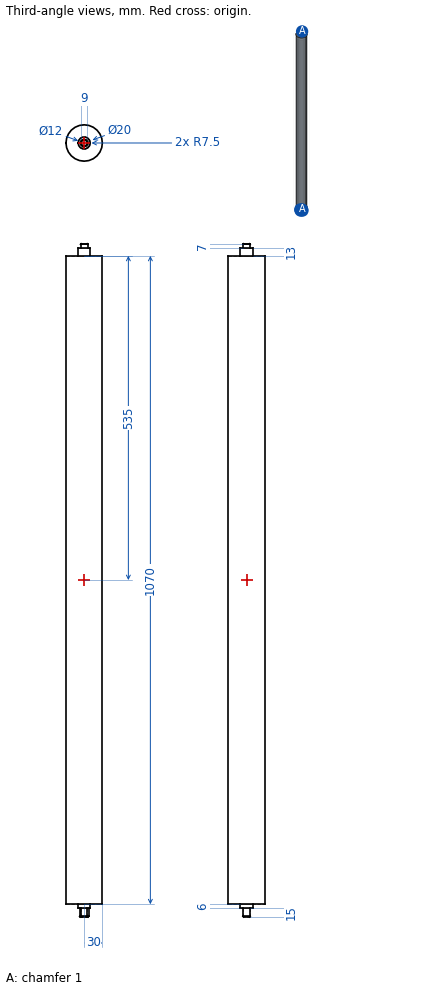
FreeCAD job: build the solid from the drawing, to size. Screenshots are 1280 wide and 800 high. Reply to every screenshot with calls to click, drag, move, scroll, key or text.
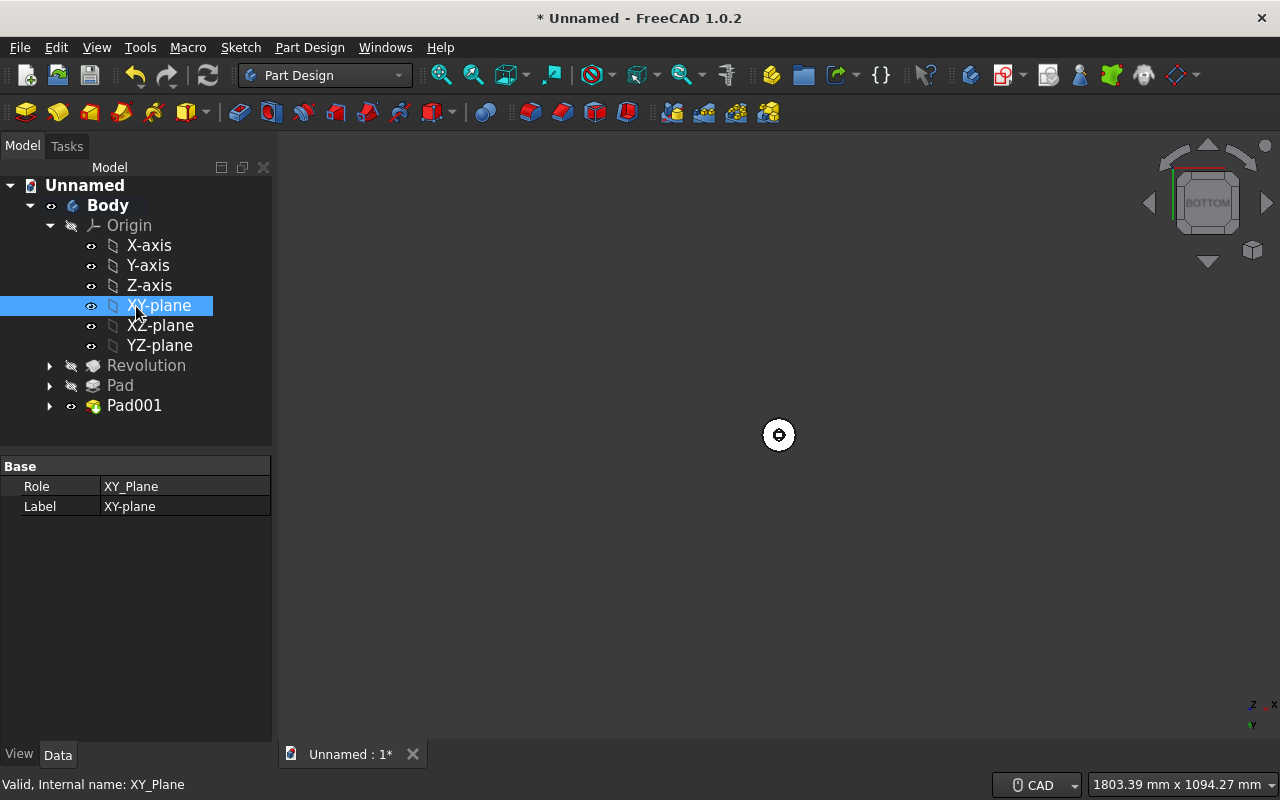
click(1176, 76)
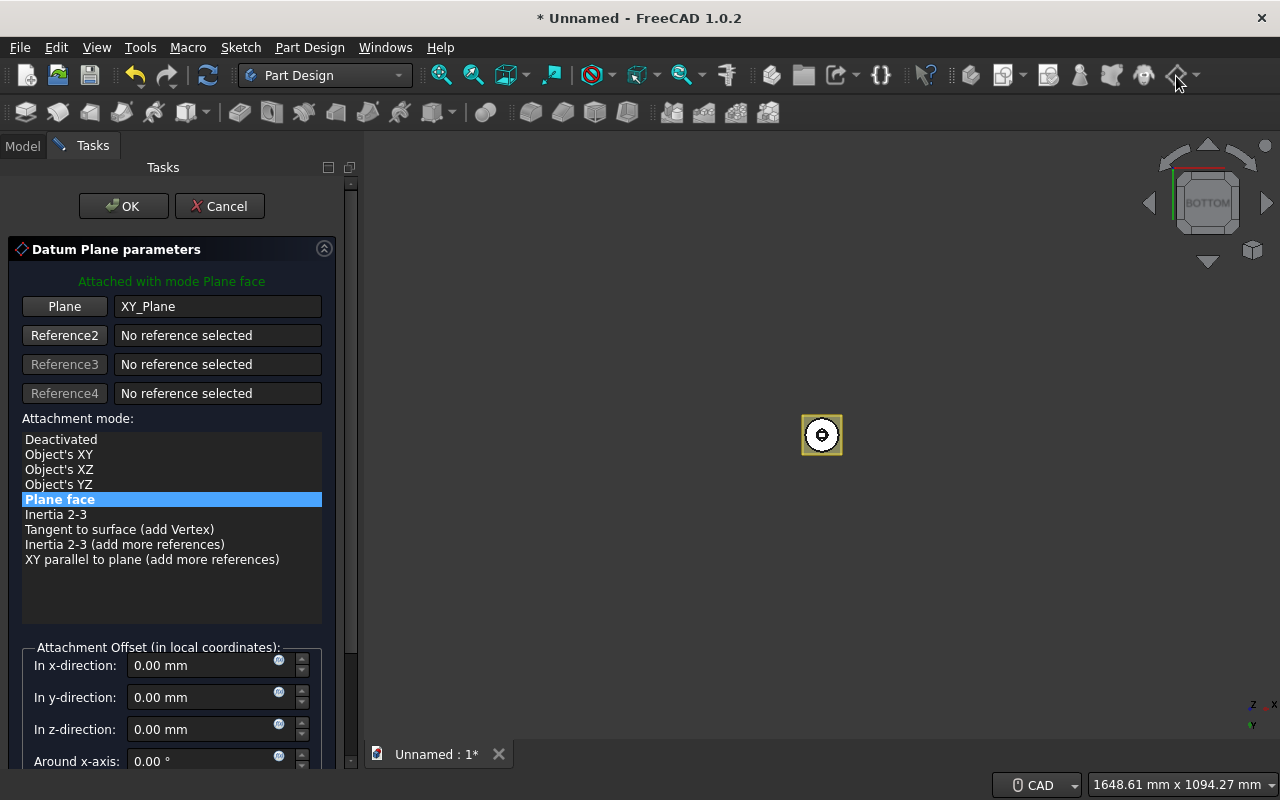
triple_click(210, 729)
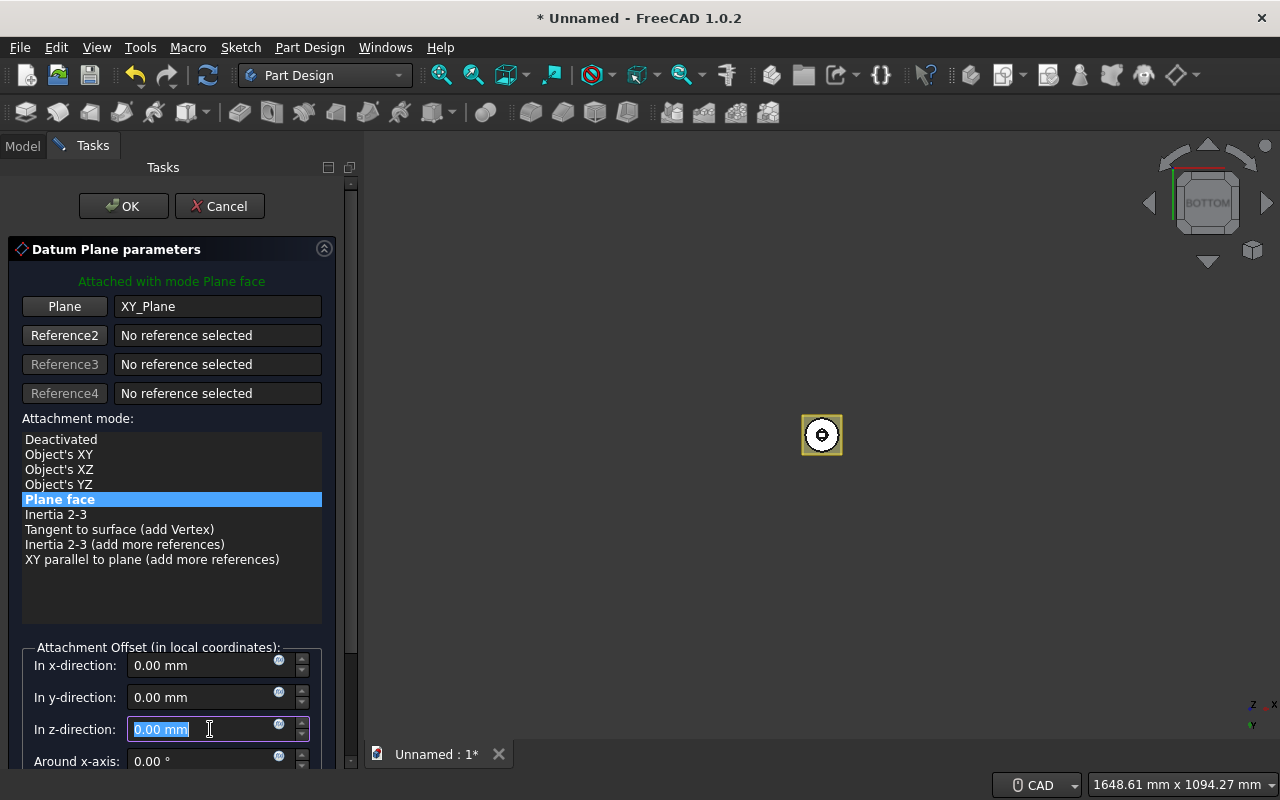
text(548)
key(Tab)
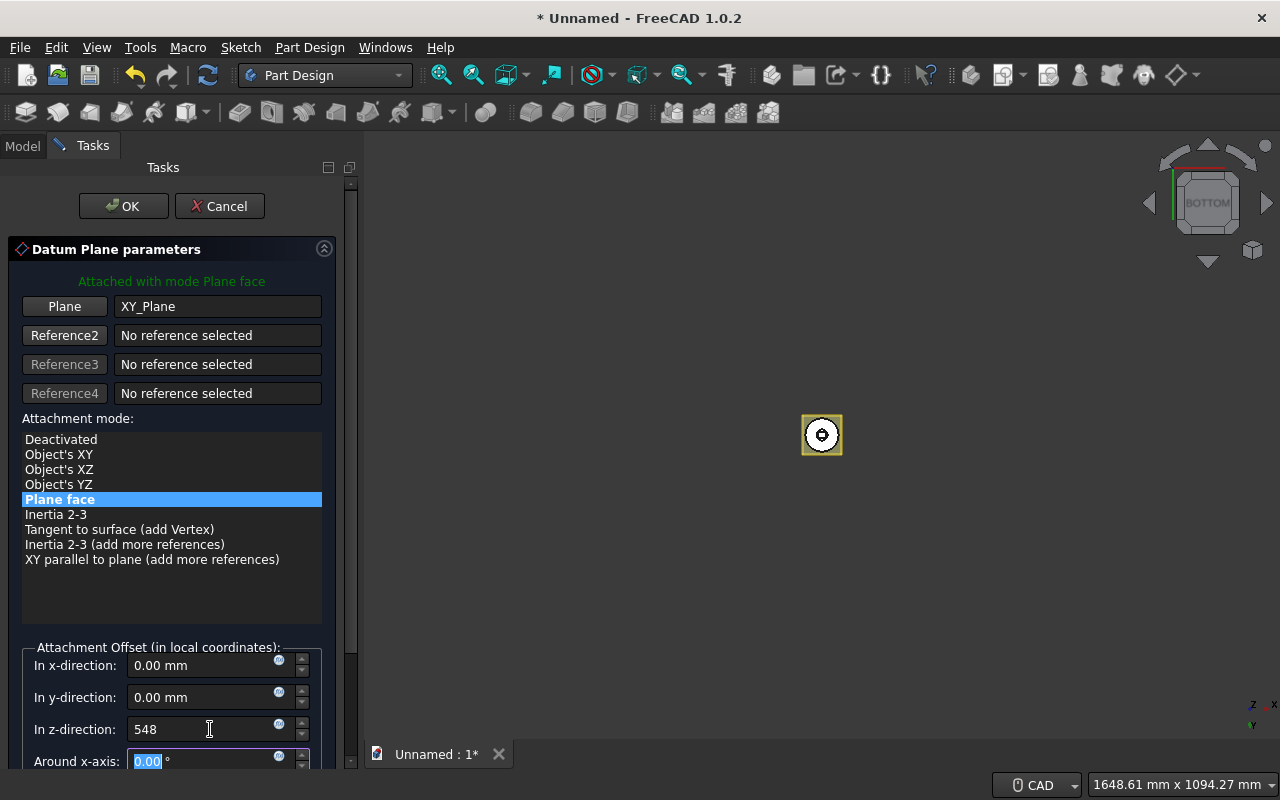
click(124, 206)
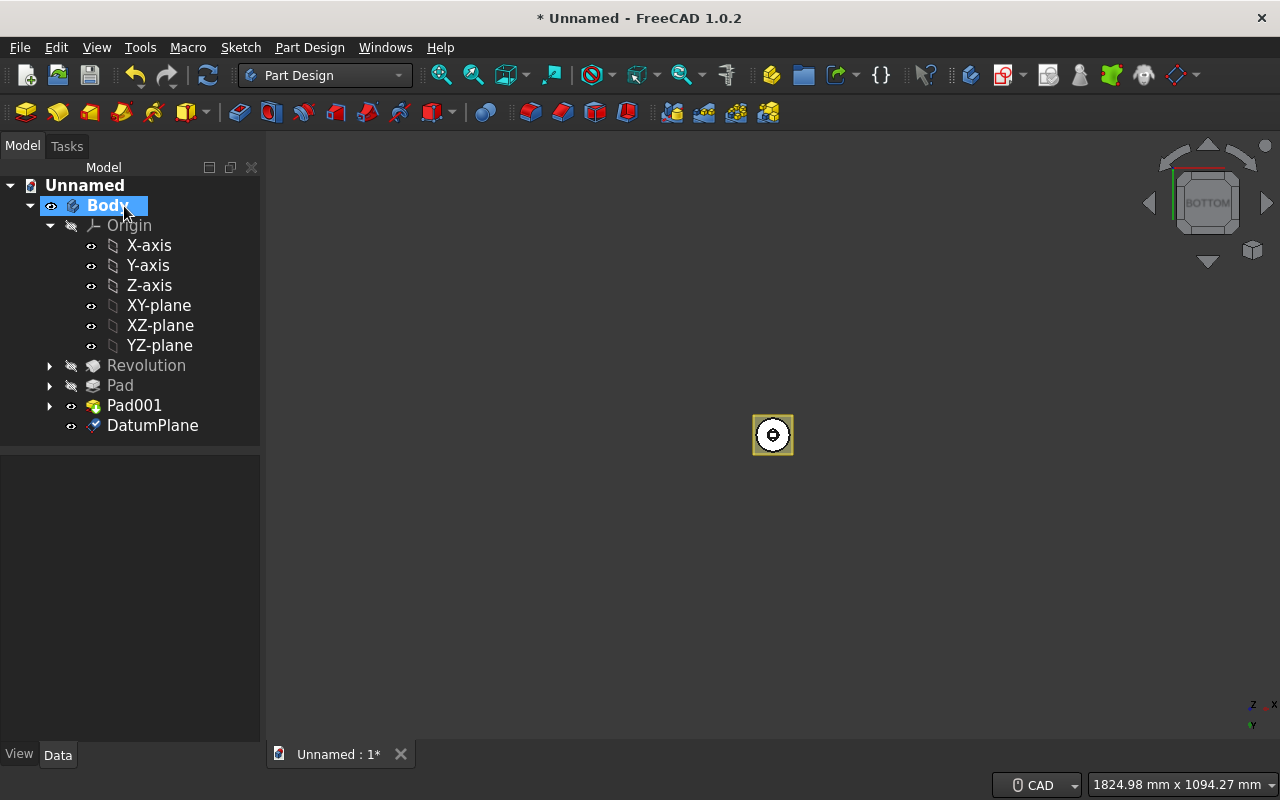
click(116, 426)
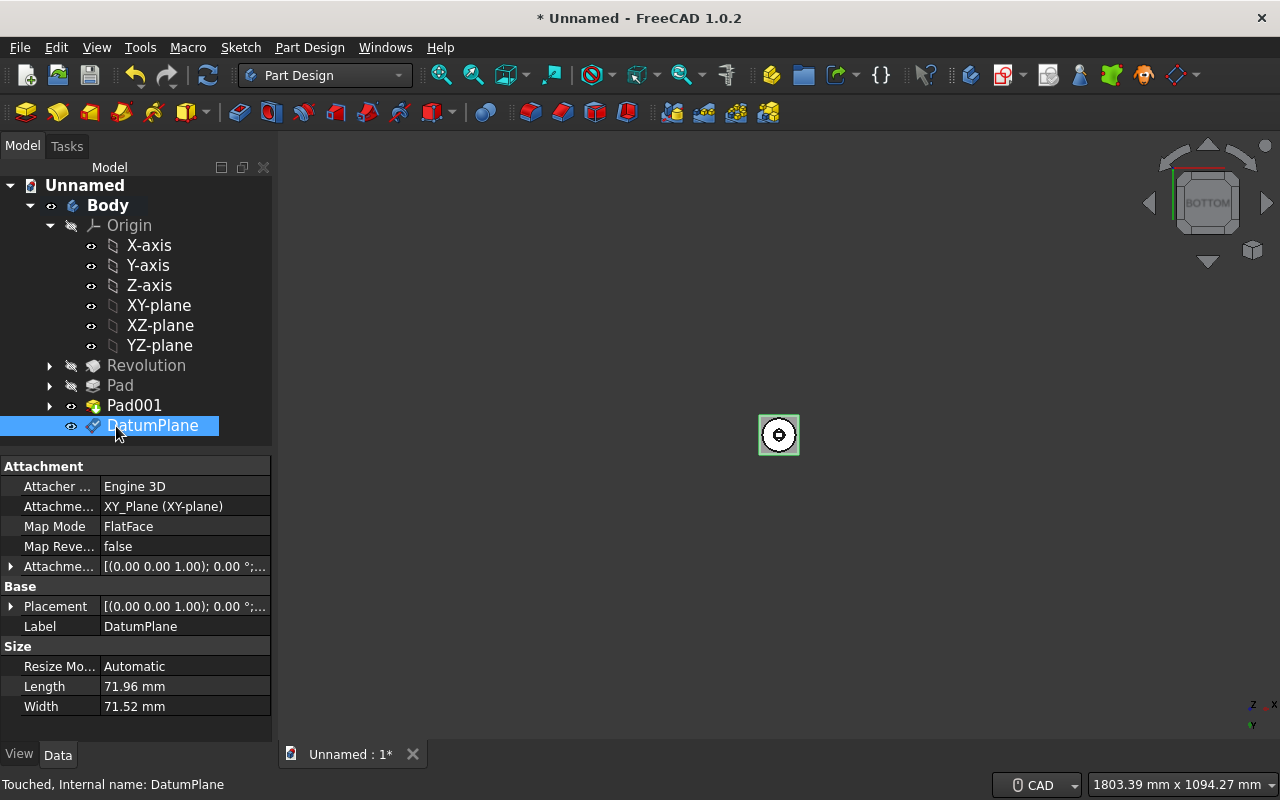
click(1004, 76)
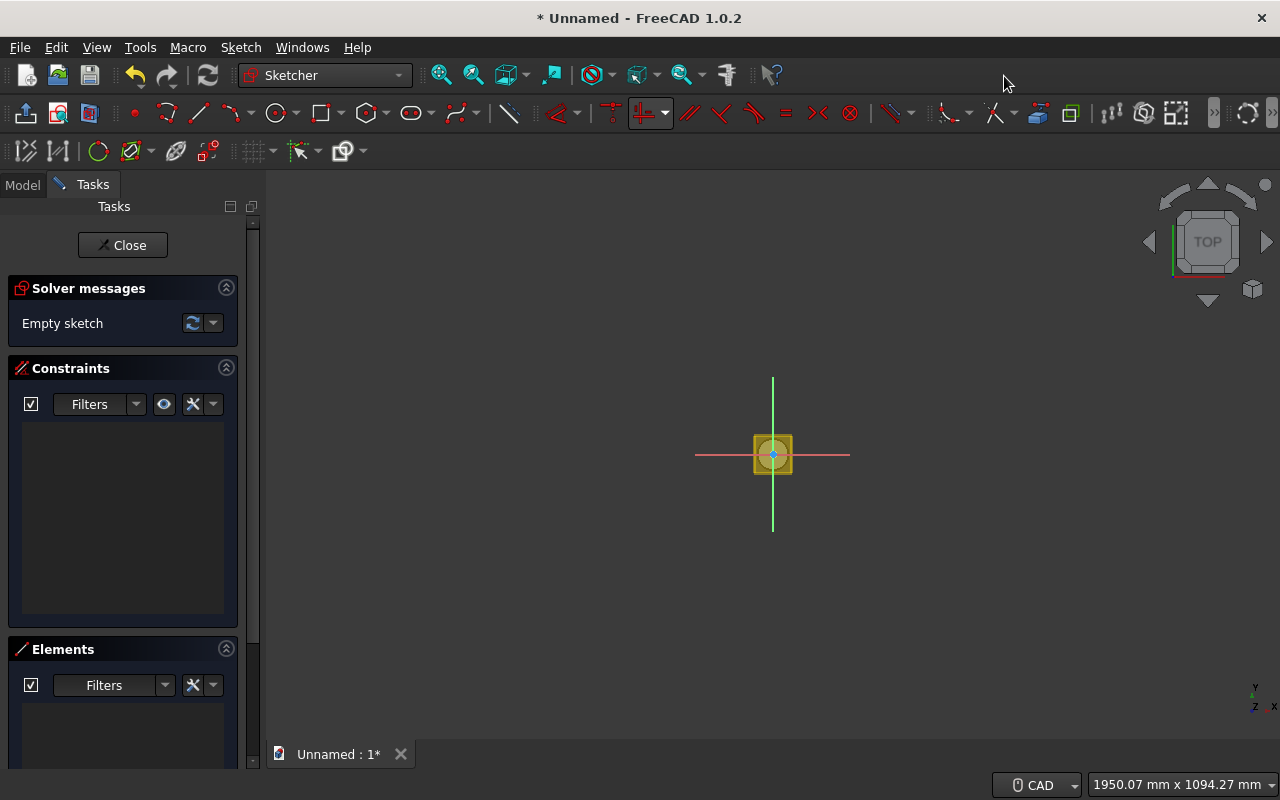
scroll(777, 455, up, 15)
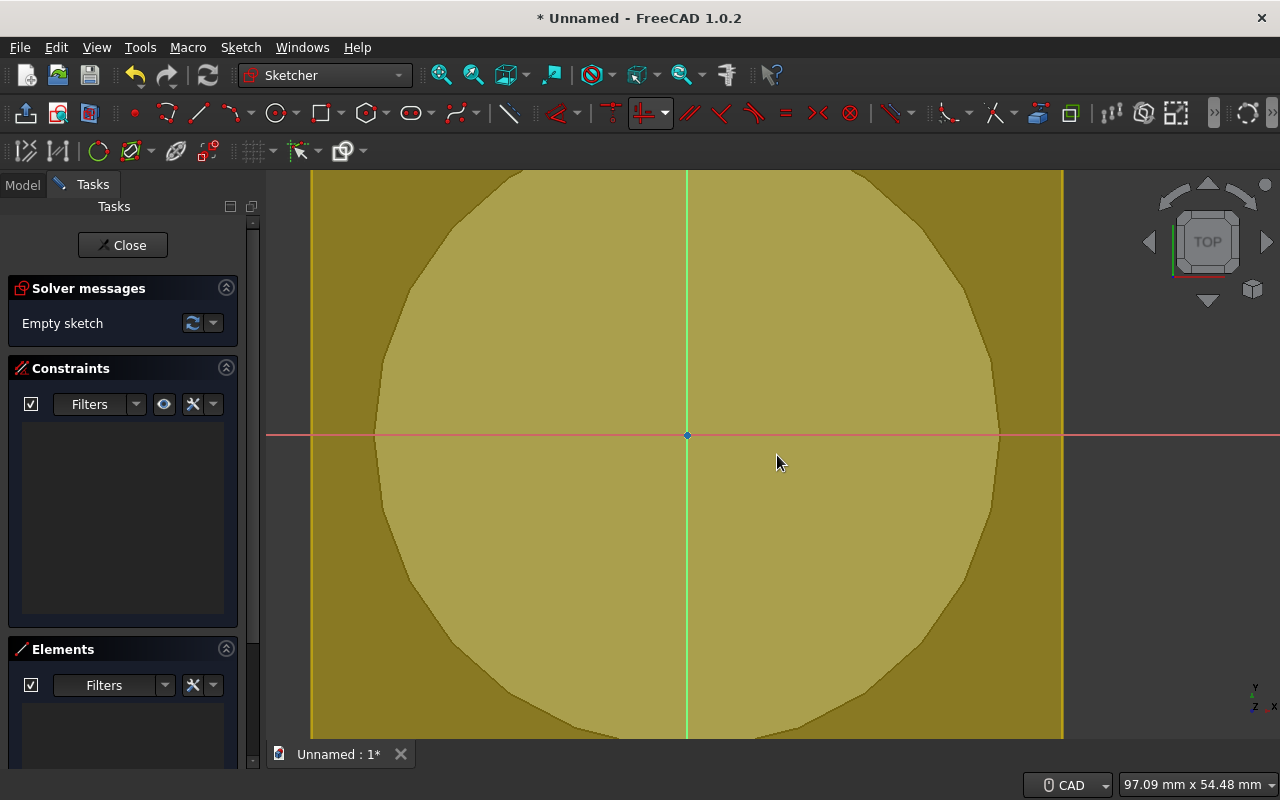
scroll(666, 412, up, 3)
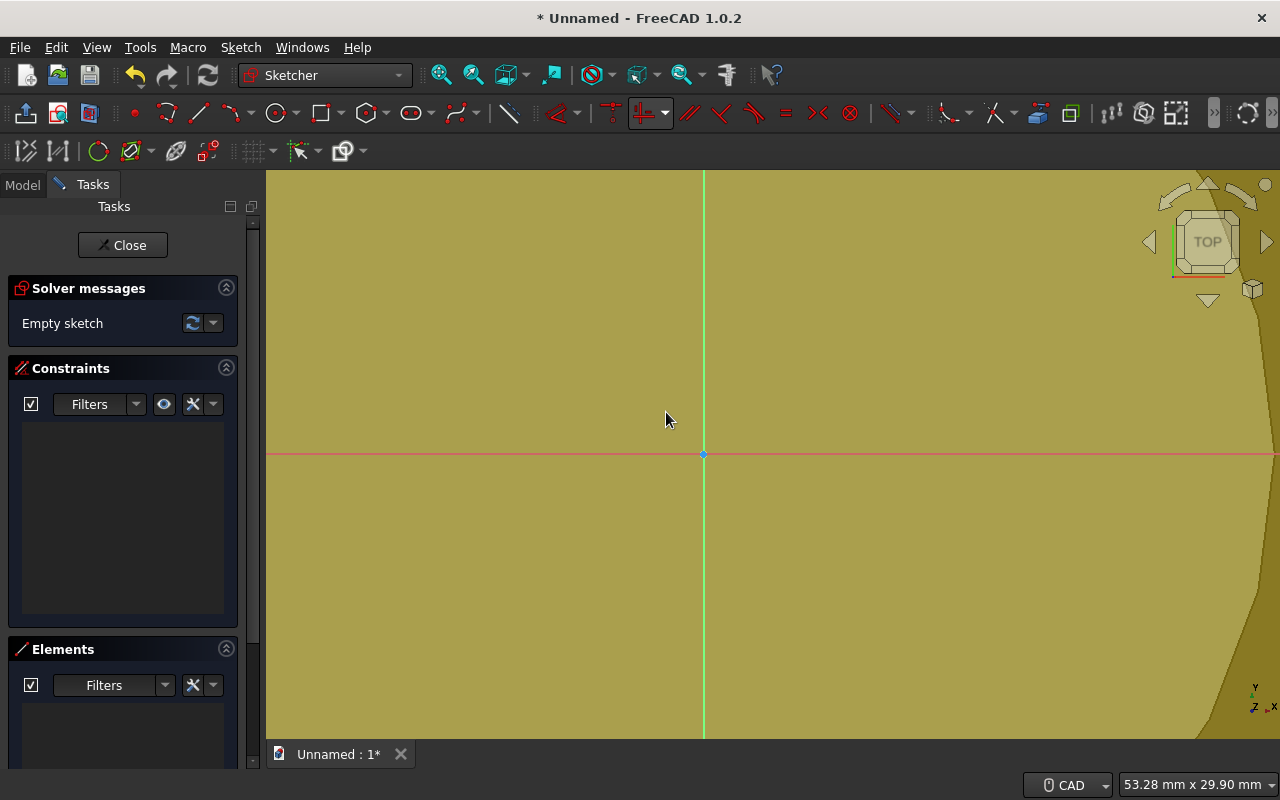
key(g)
key(c)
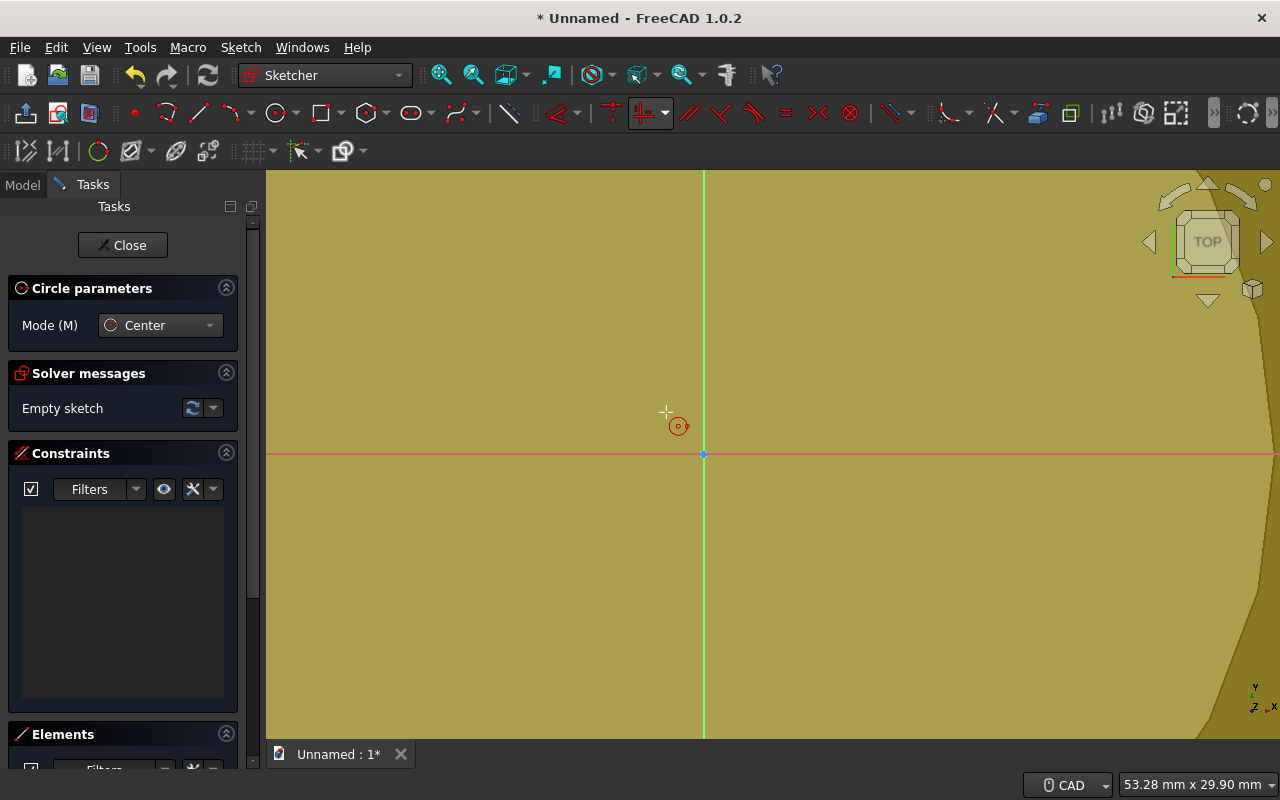
click(704, 454)
move(839, 320)